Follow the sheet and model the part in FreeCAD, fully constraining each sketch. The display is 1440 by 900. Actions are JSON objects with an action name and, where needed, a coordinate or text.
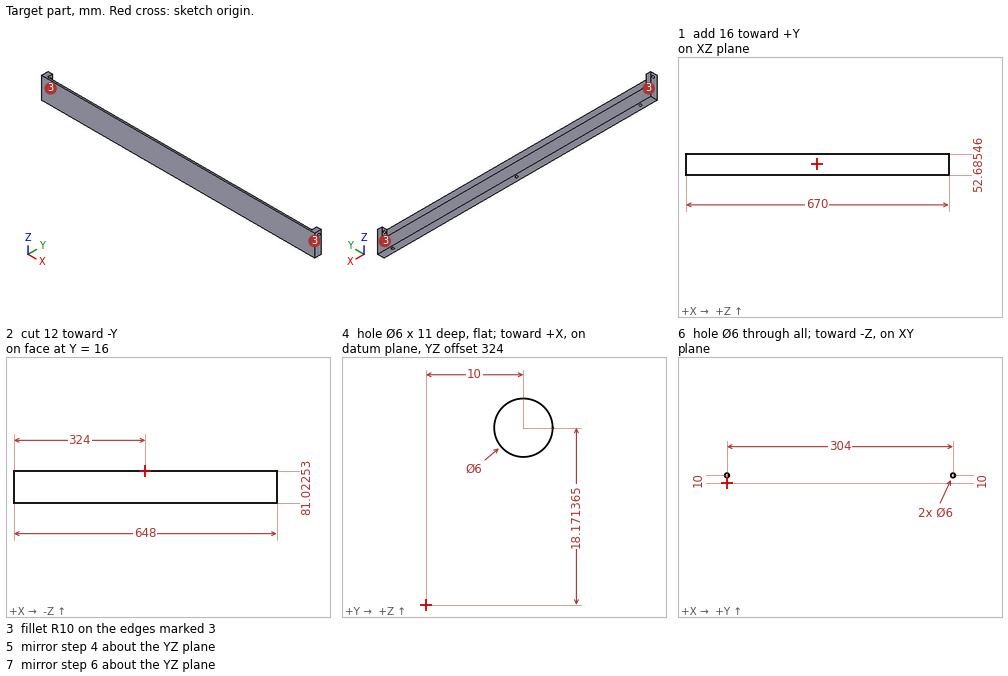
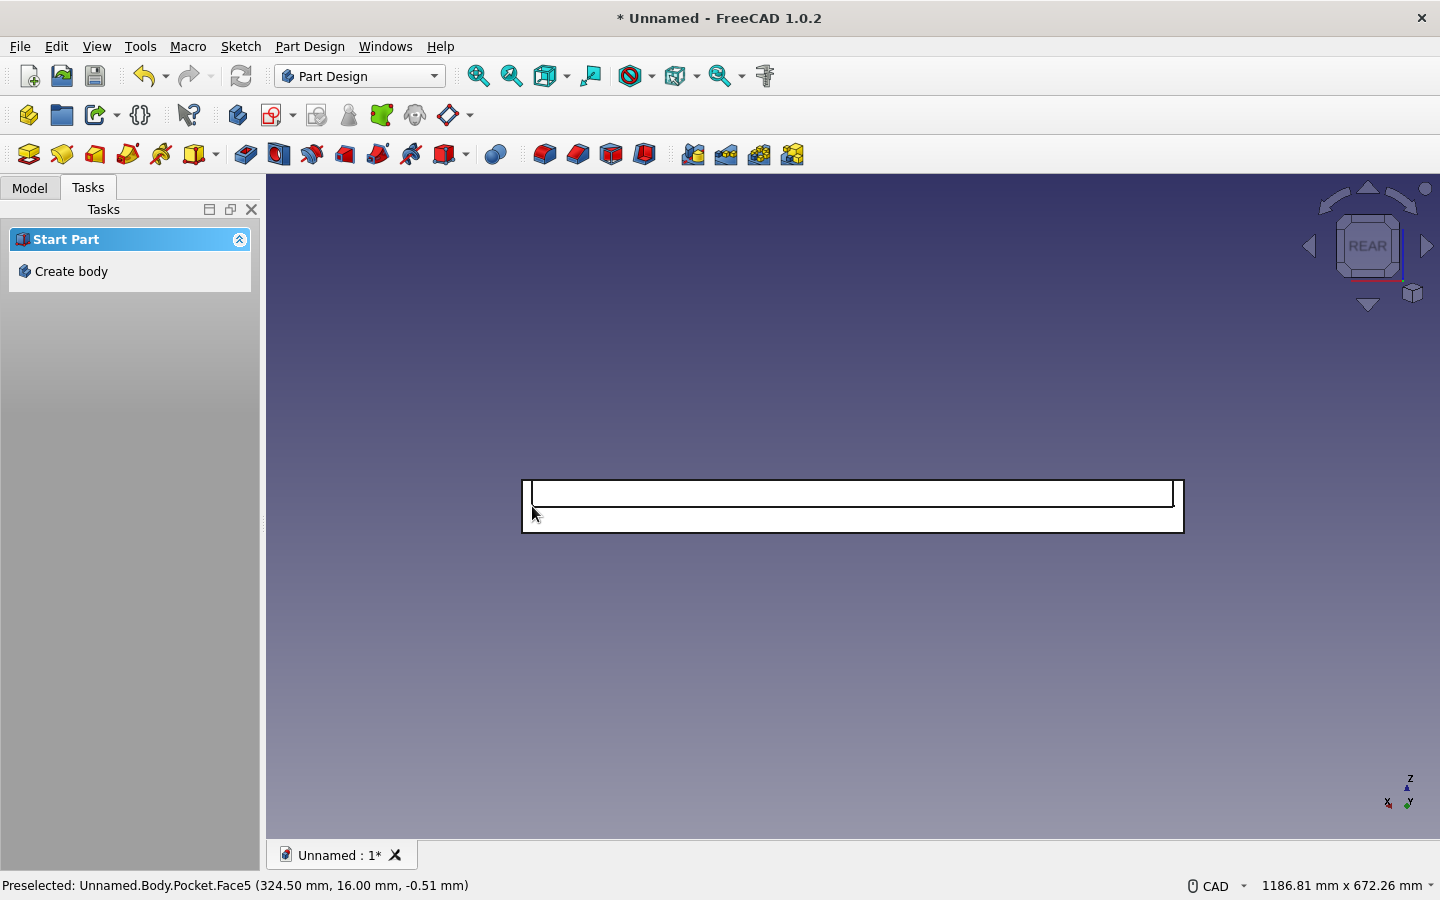
{"action": "key", "text": "0"}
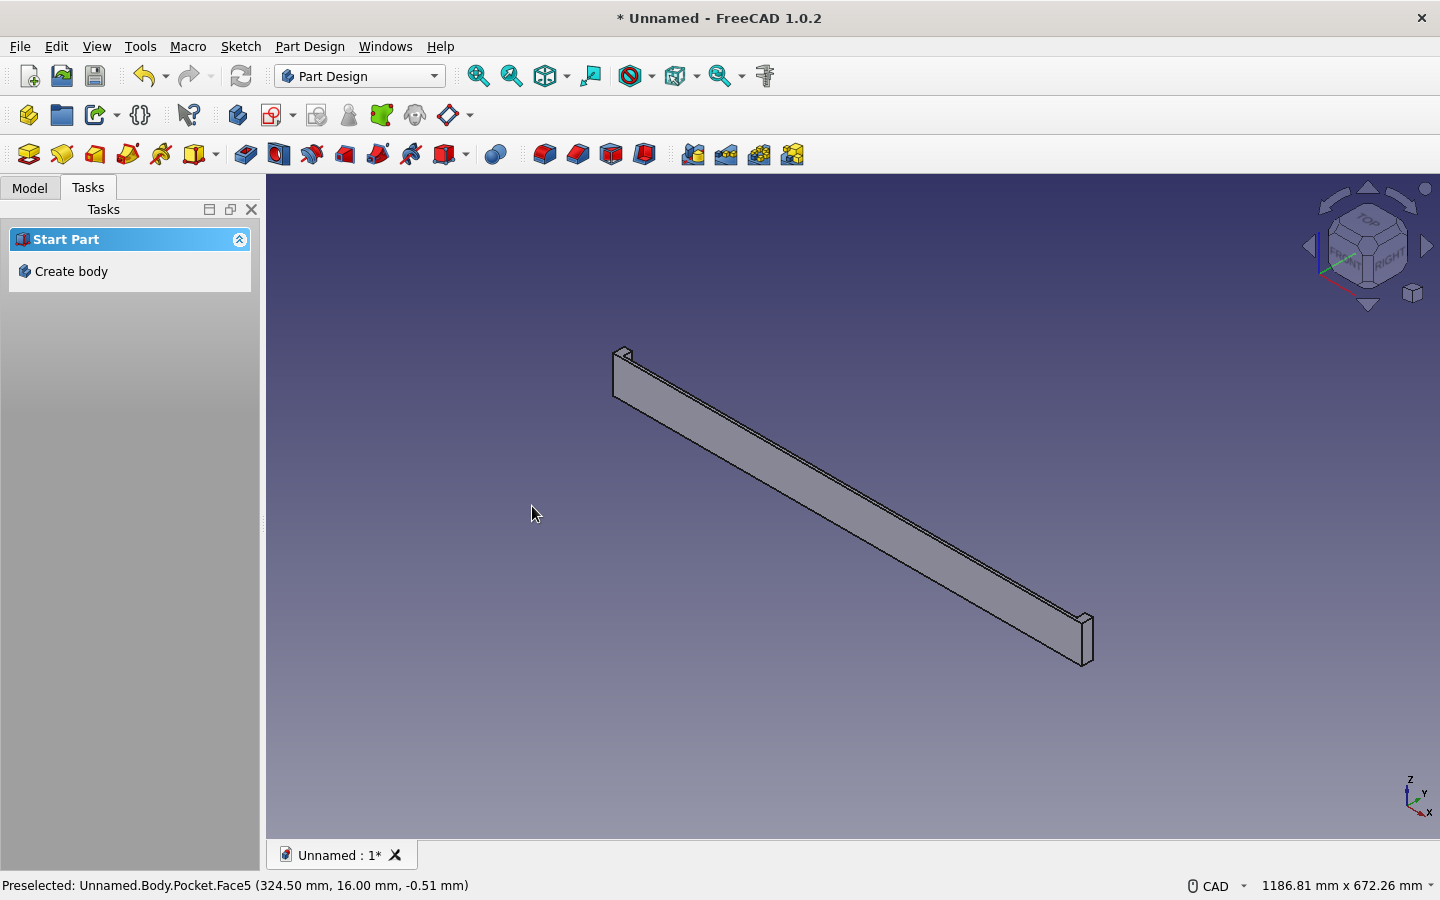
{"action": "scroll", "coordinate": [1081, 636], "scroll_direction": "up", "scroll_amount": 7}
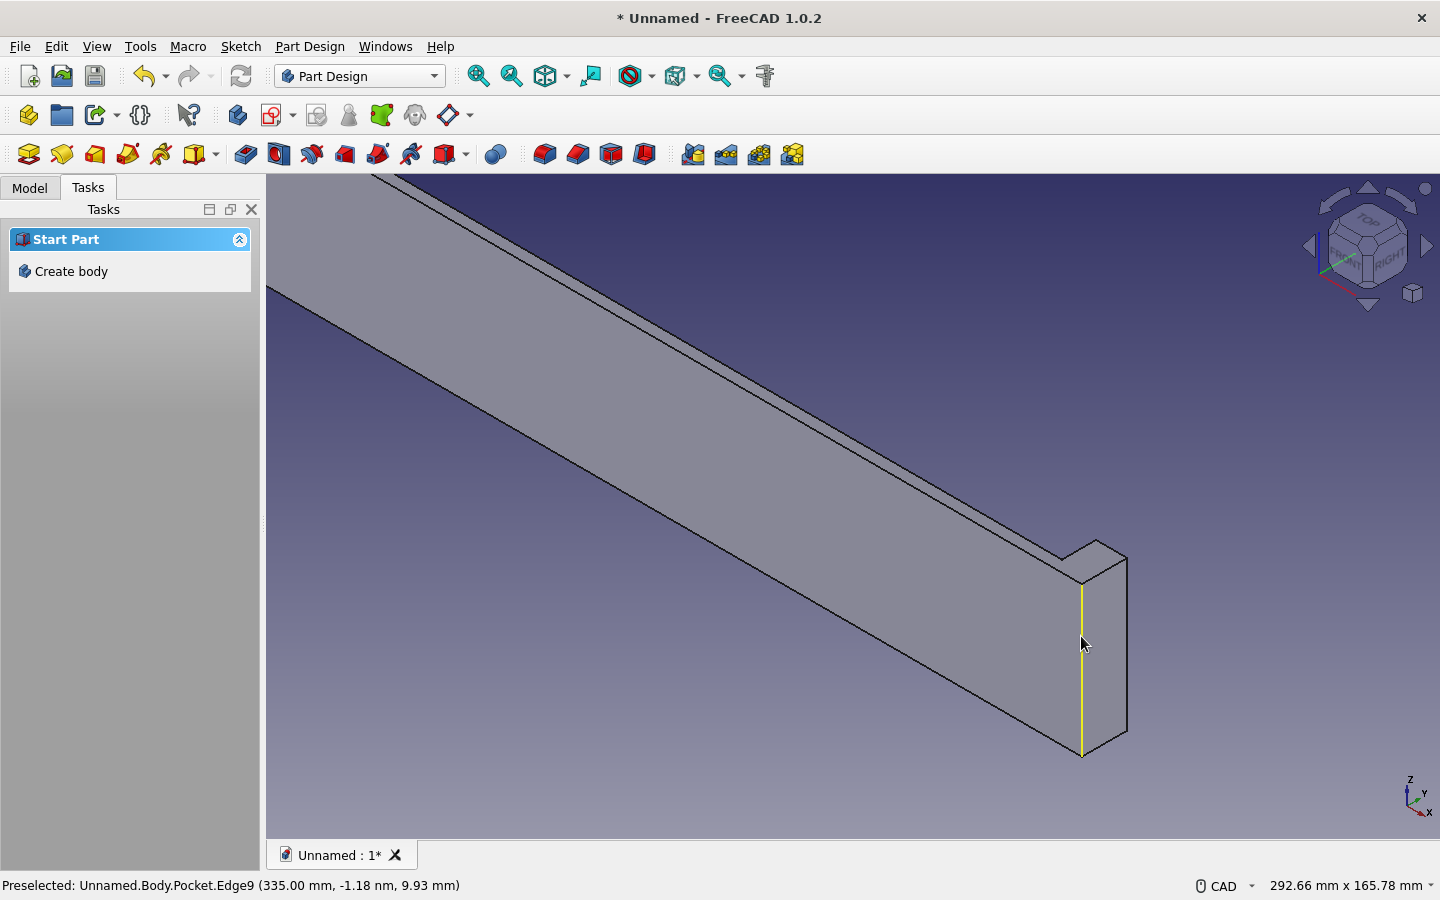
{"action": "left_click", "coordinate": [479, 76]}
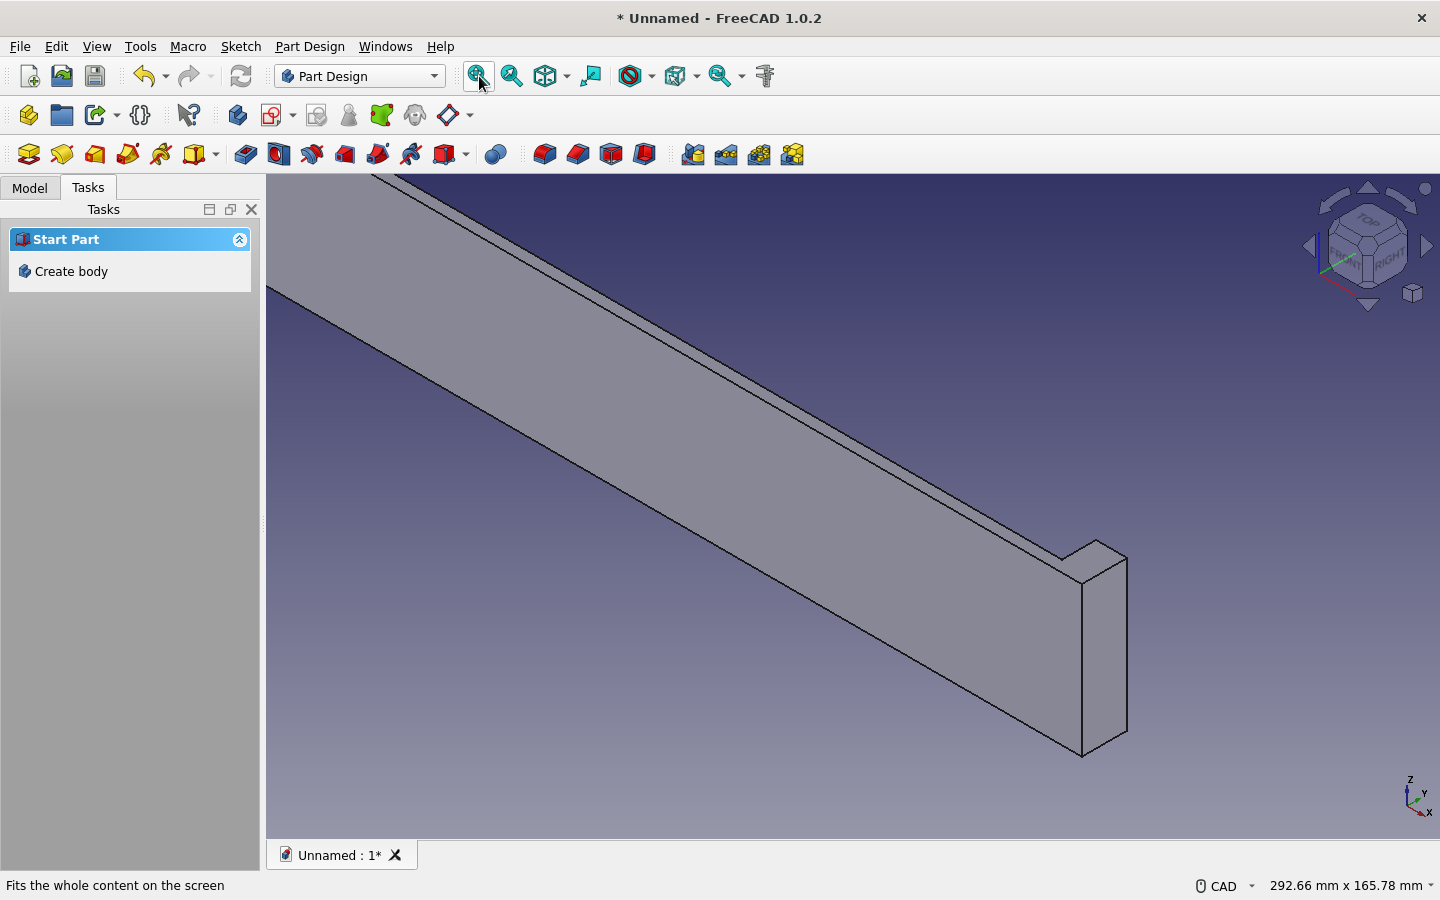
{"action": "key", "text": "2"}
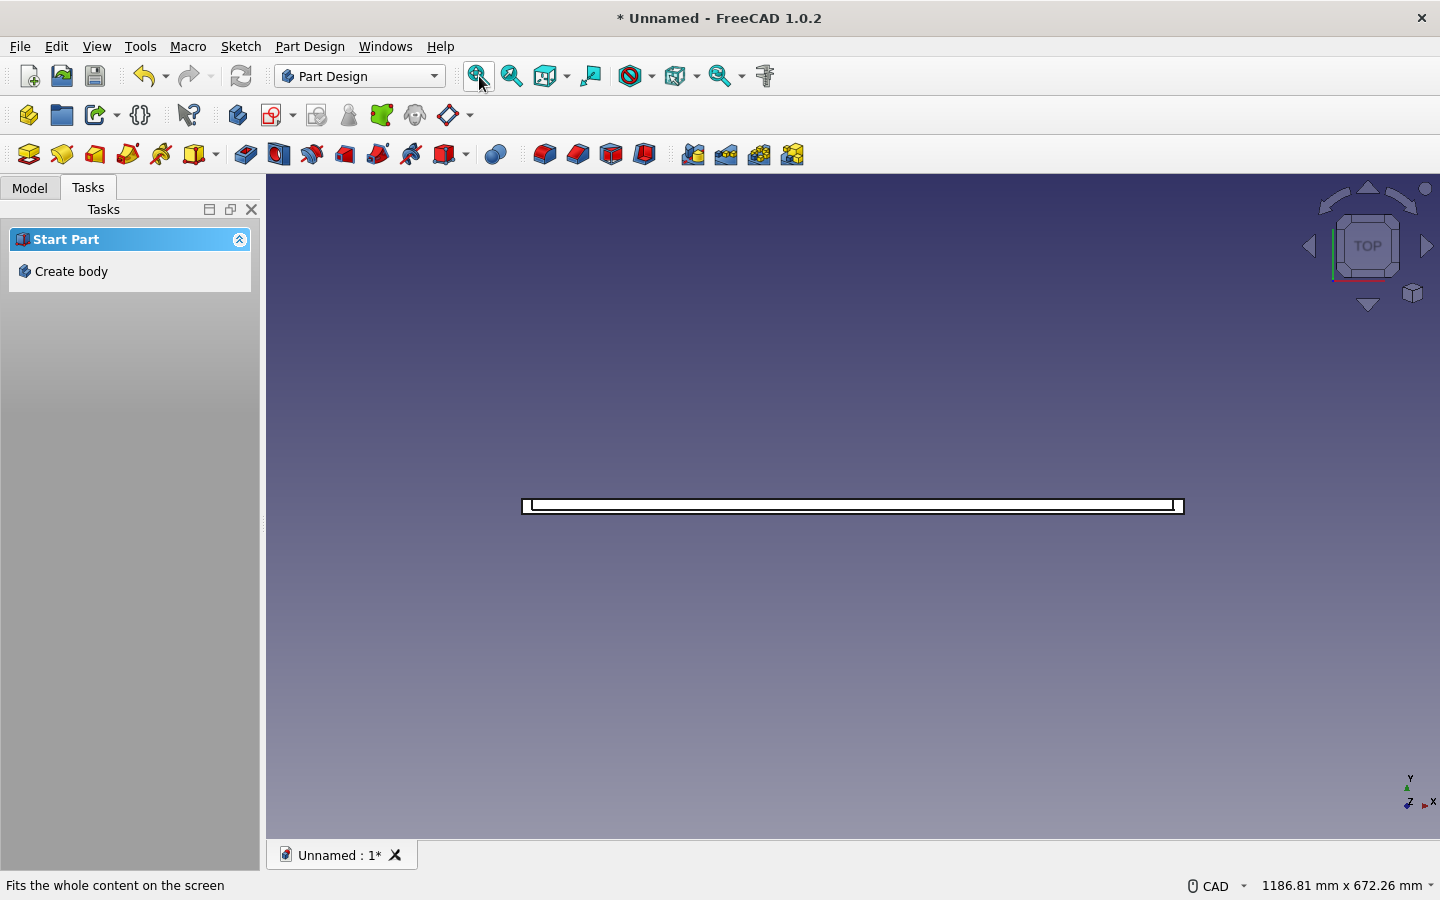
{"action": "scroll", "coordinate": [1174, 504], "scroll_direction": "up", "scroll_amount": 7}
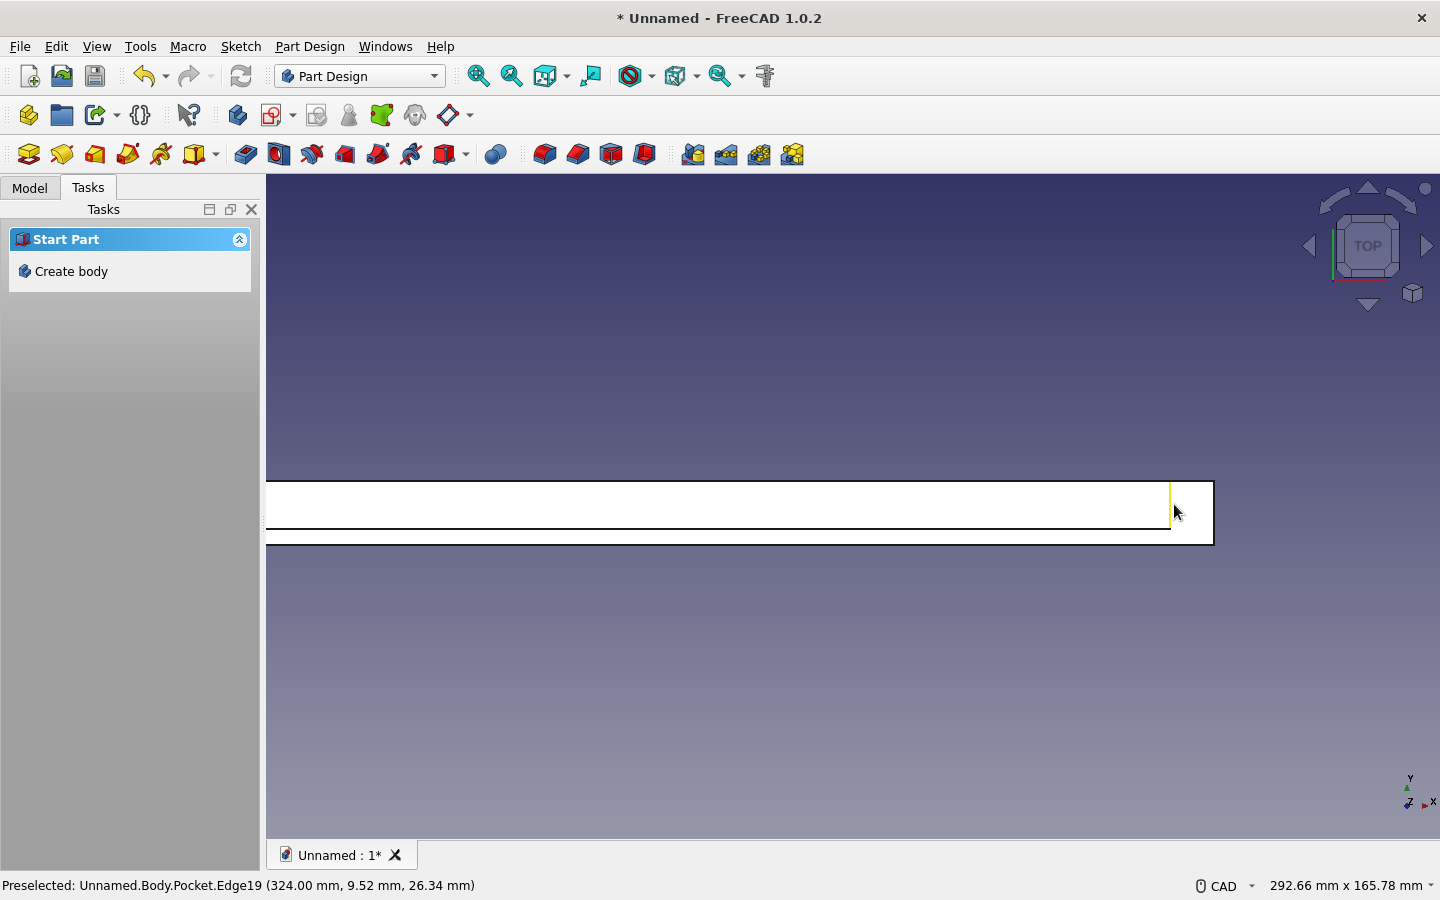
{"action": "key", "text": "v f"}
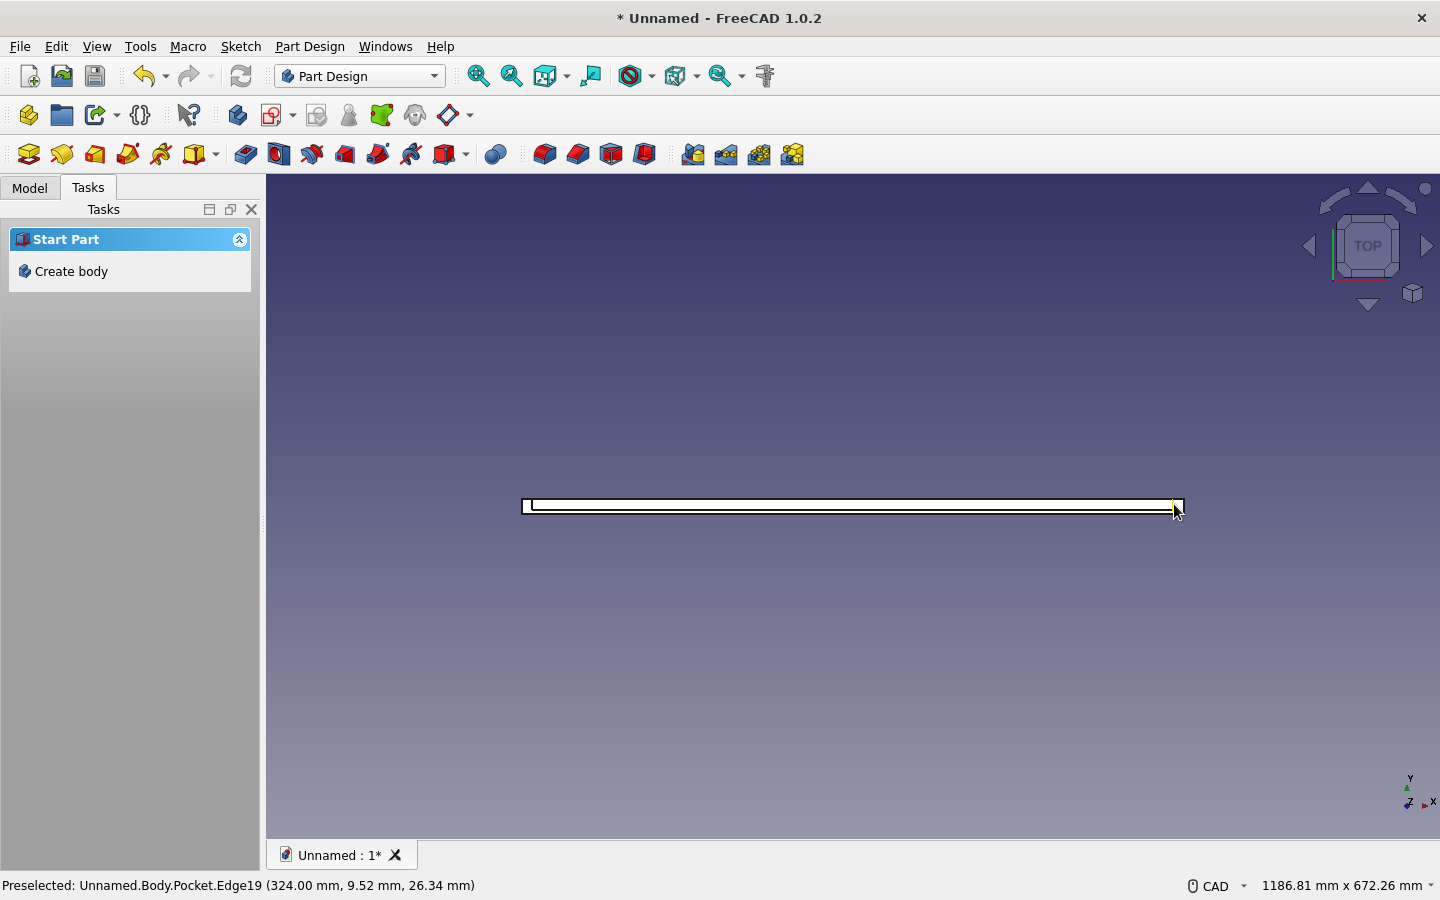
{"action": "key", "text": "1"}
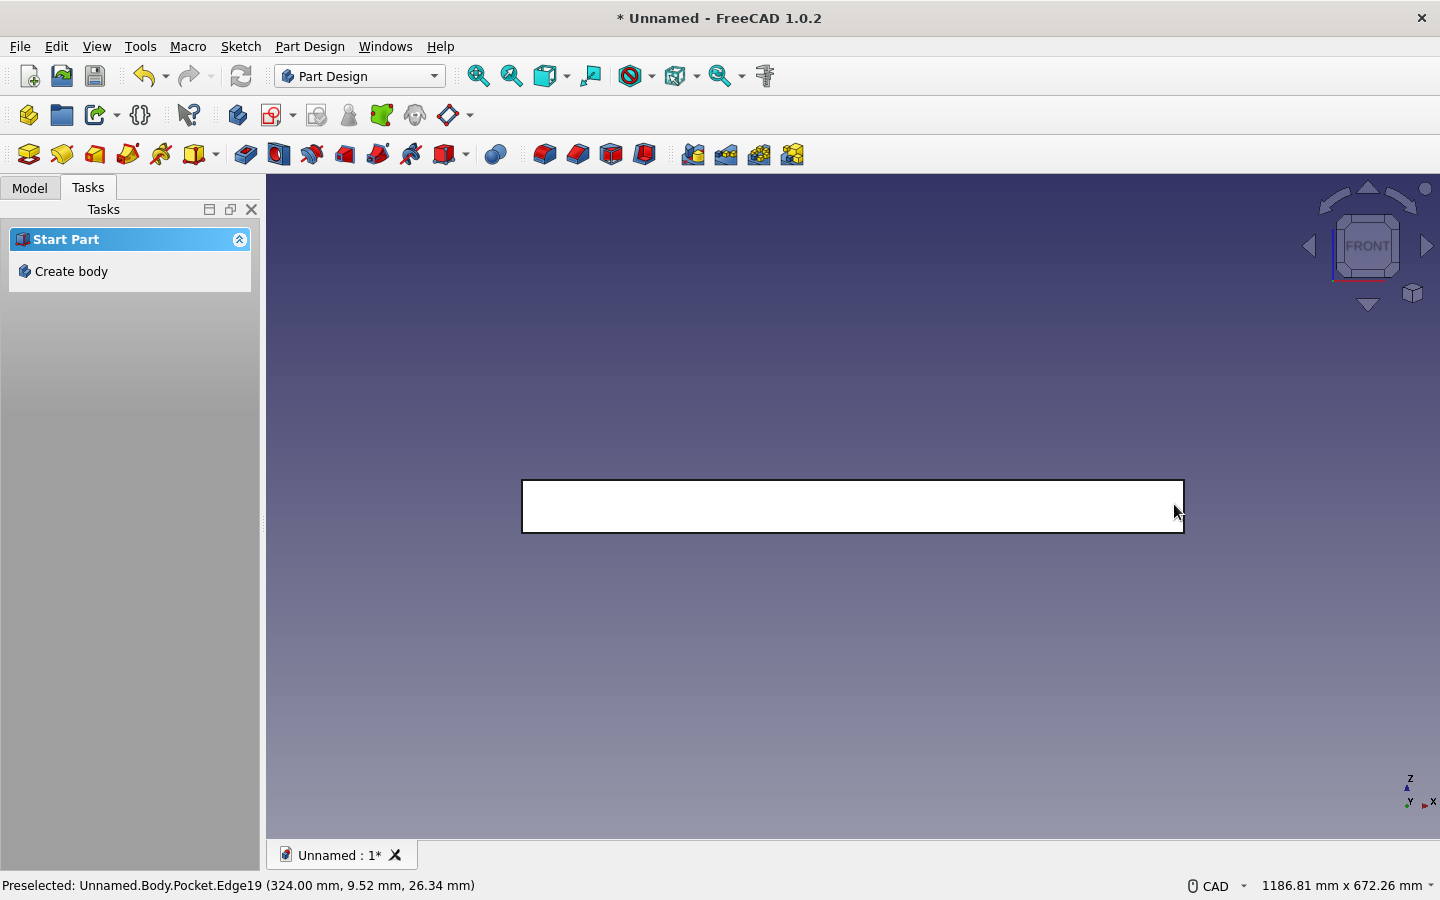
{"action": "scroll", "coordinate": [1174, 506], "scroll_direction": "up", "scroll_amount": 7}